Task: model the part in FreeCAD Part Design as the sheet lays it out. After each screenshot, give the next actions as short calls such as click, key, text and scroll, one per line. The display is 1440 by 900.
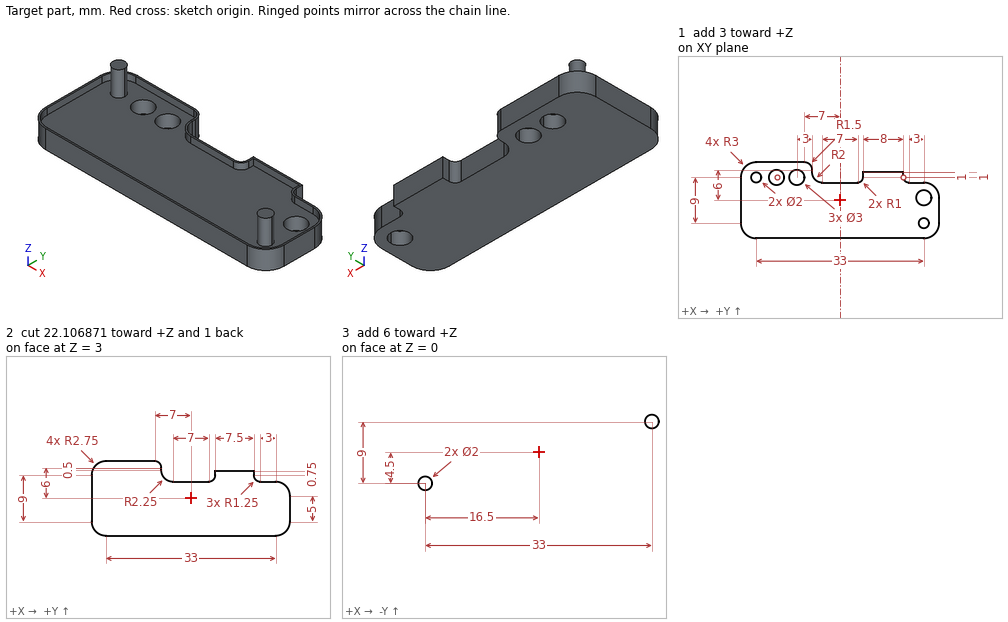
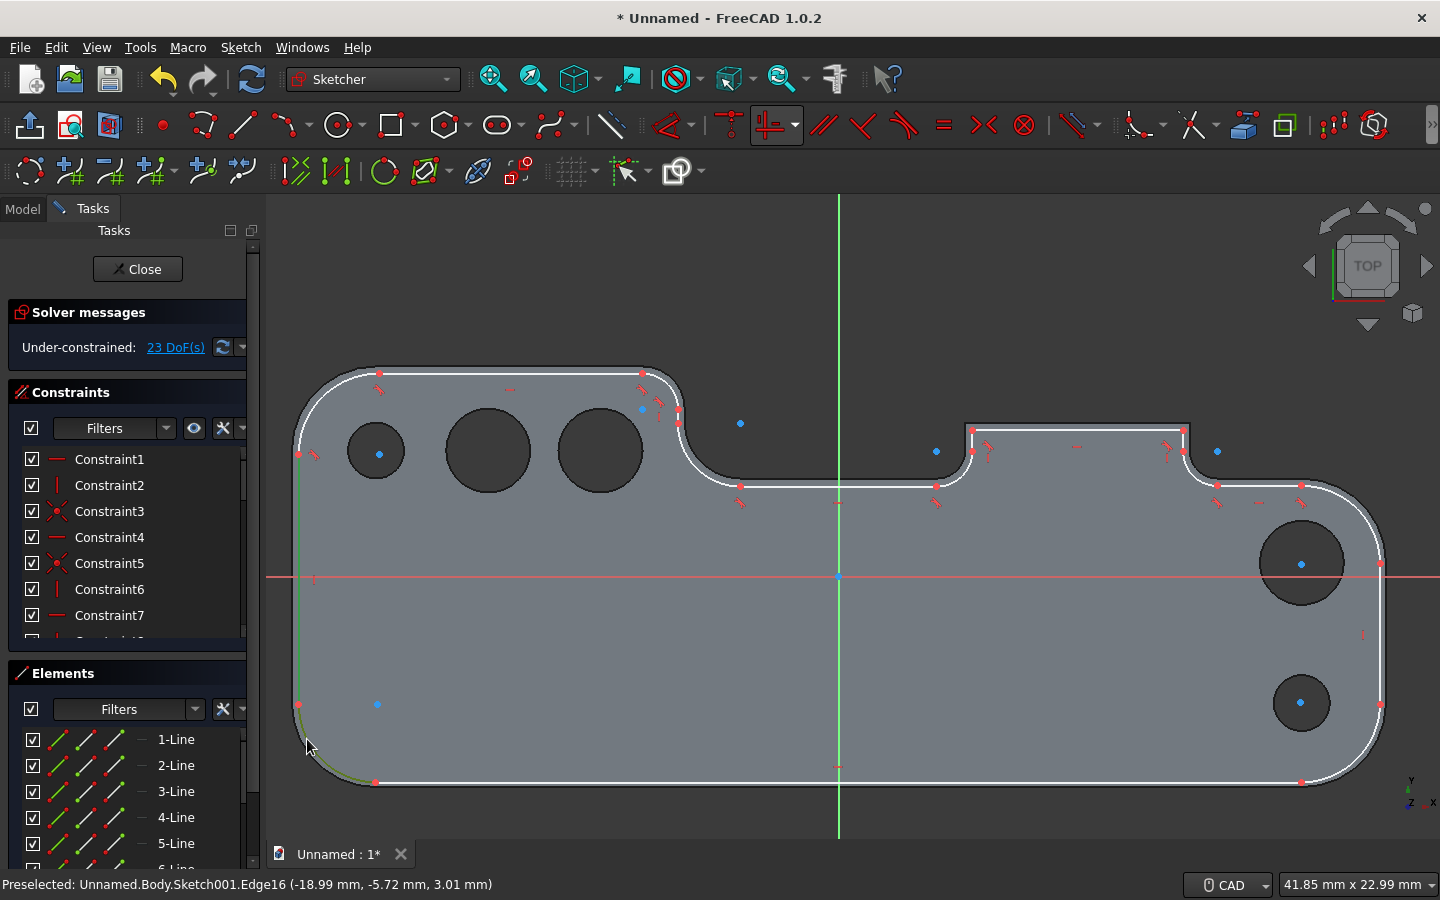
click(904, 126)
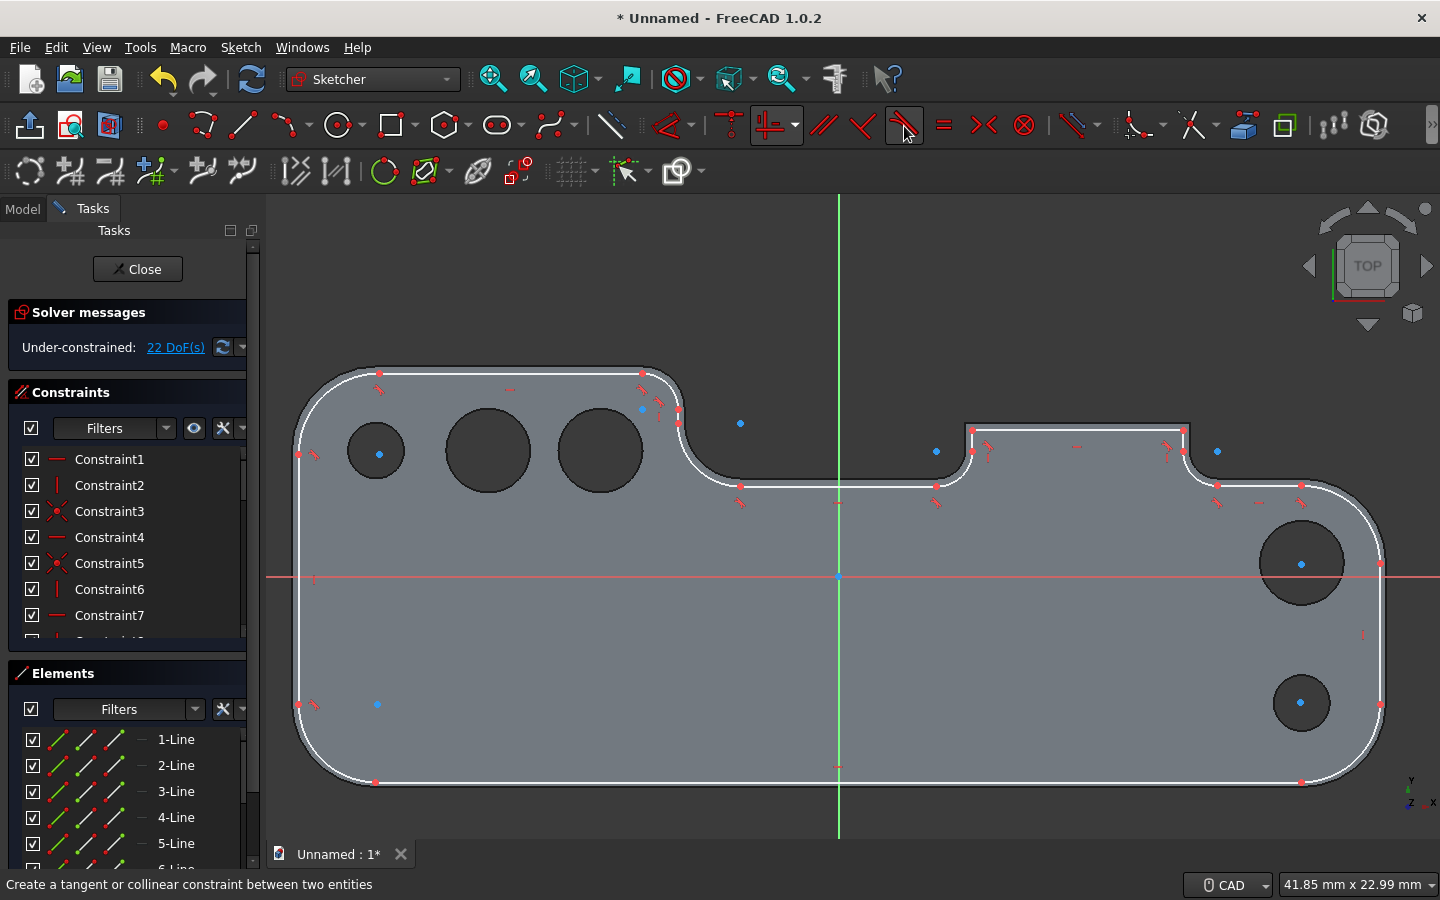
click(653, 783)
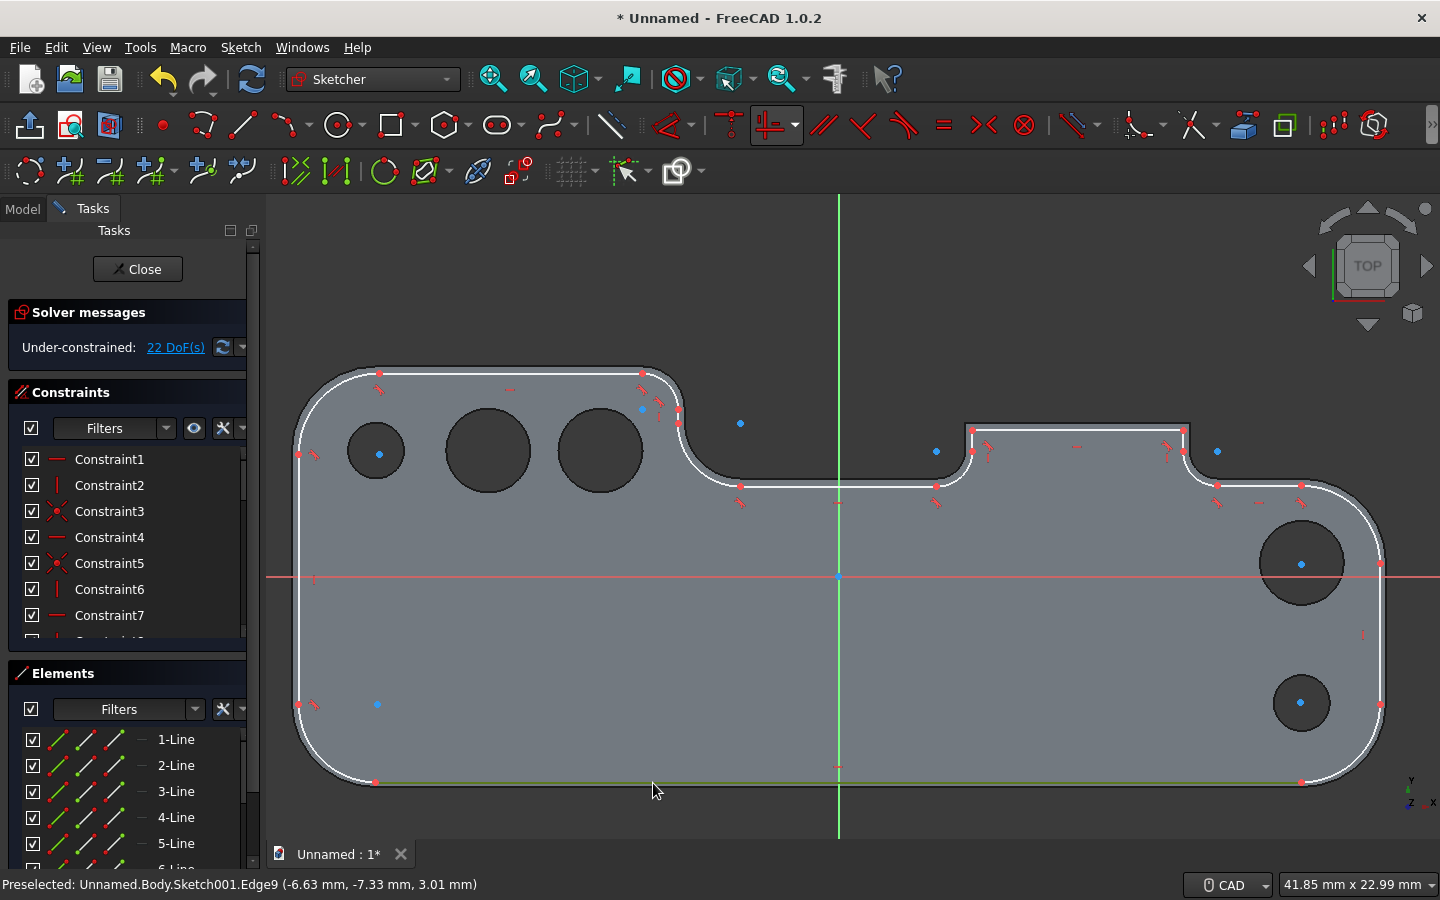
click(307, 739)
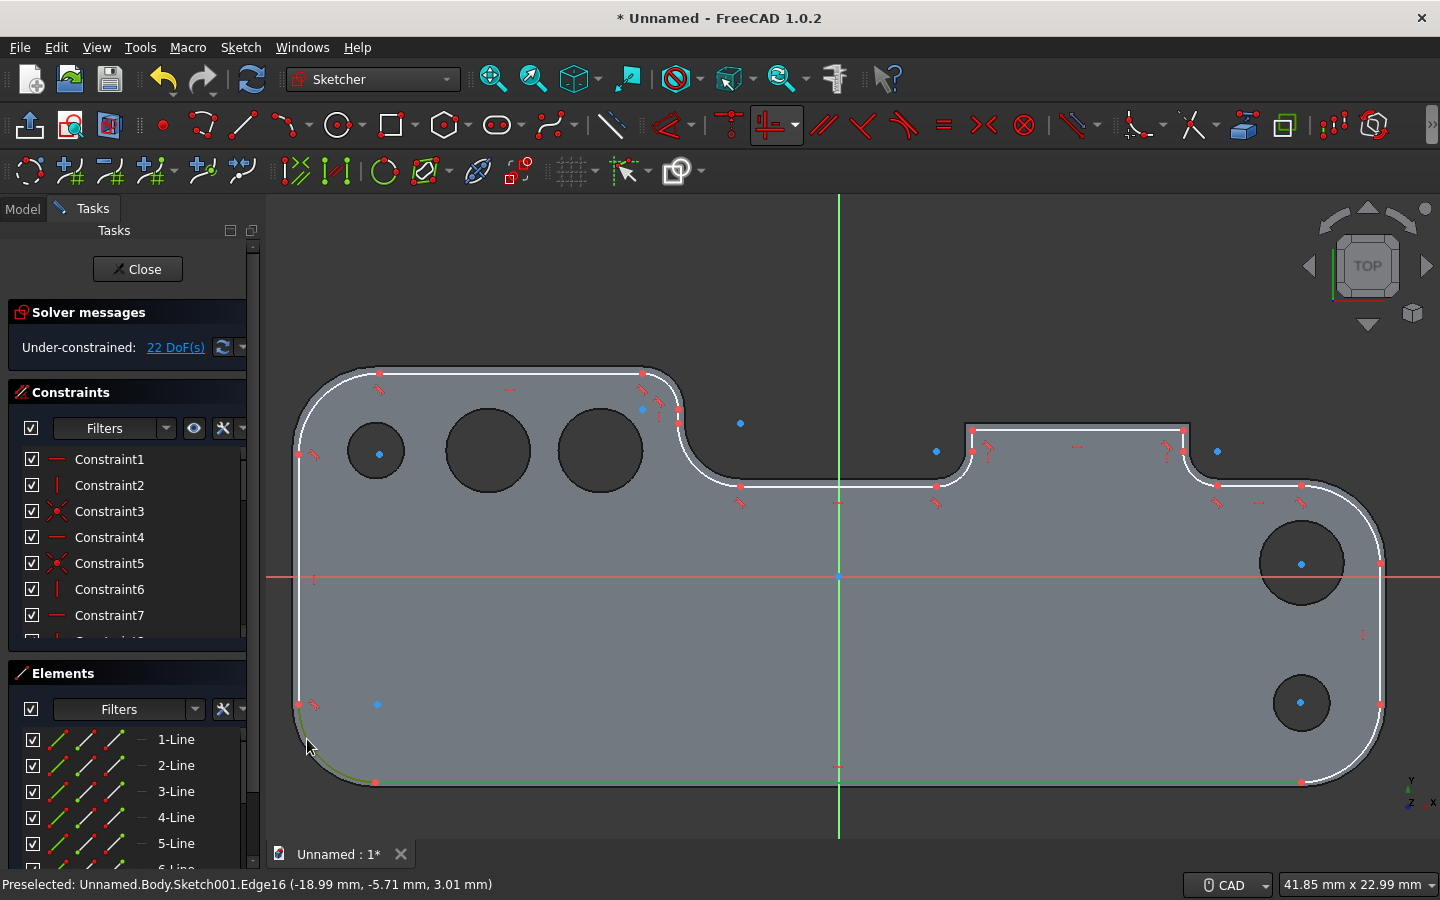
click(904, 126)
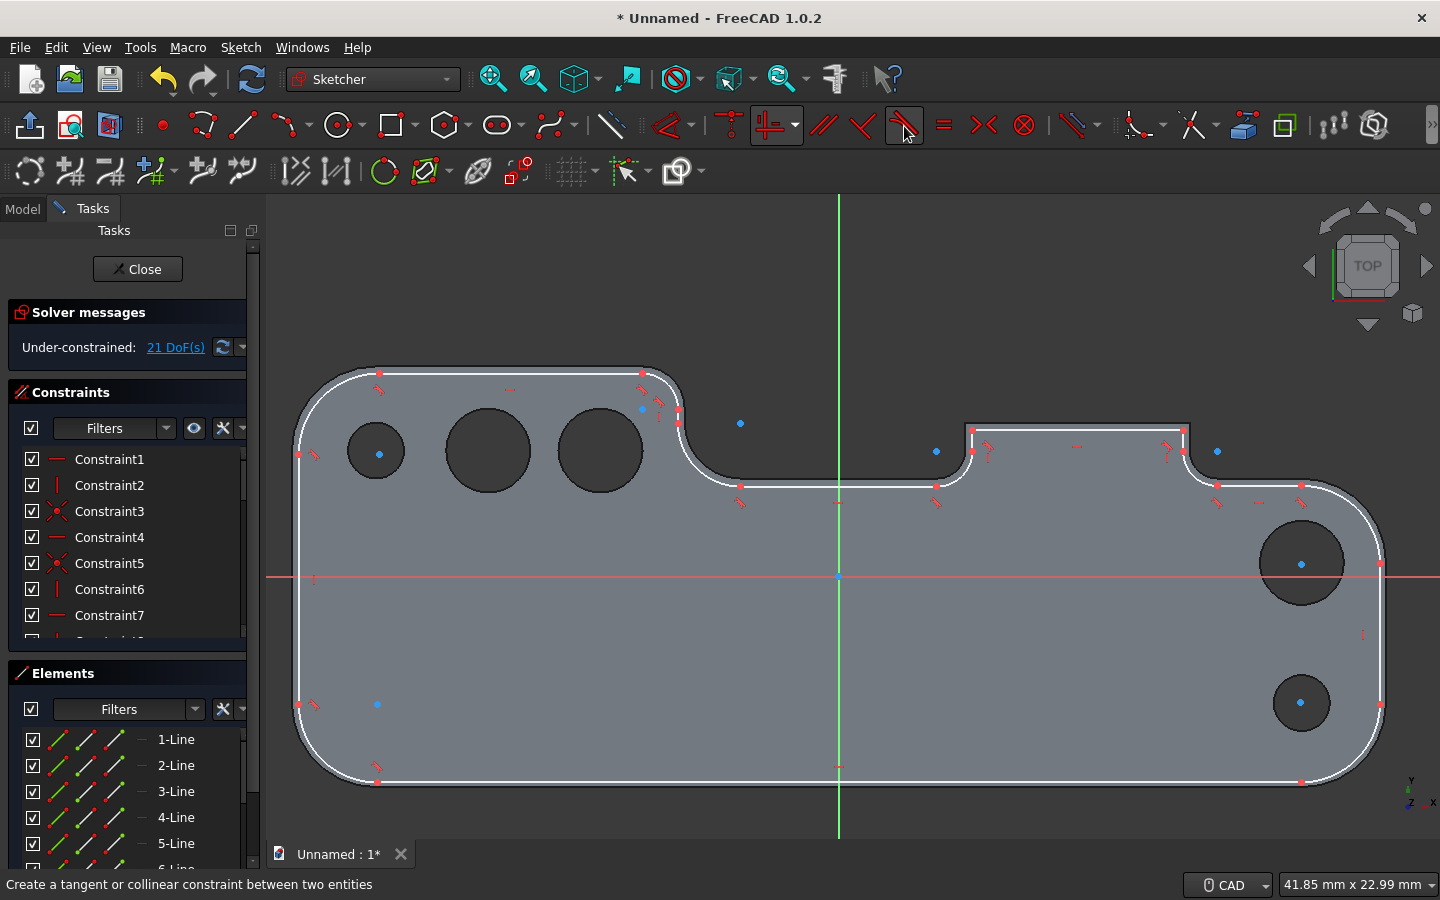
click(655, 782)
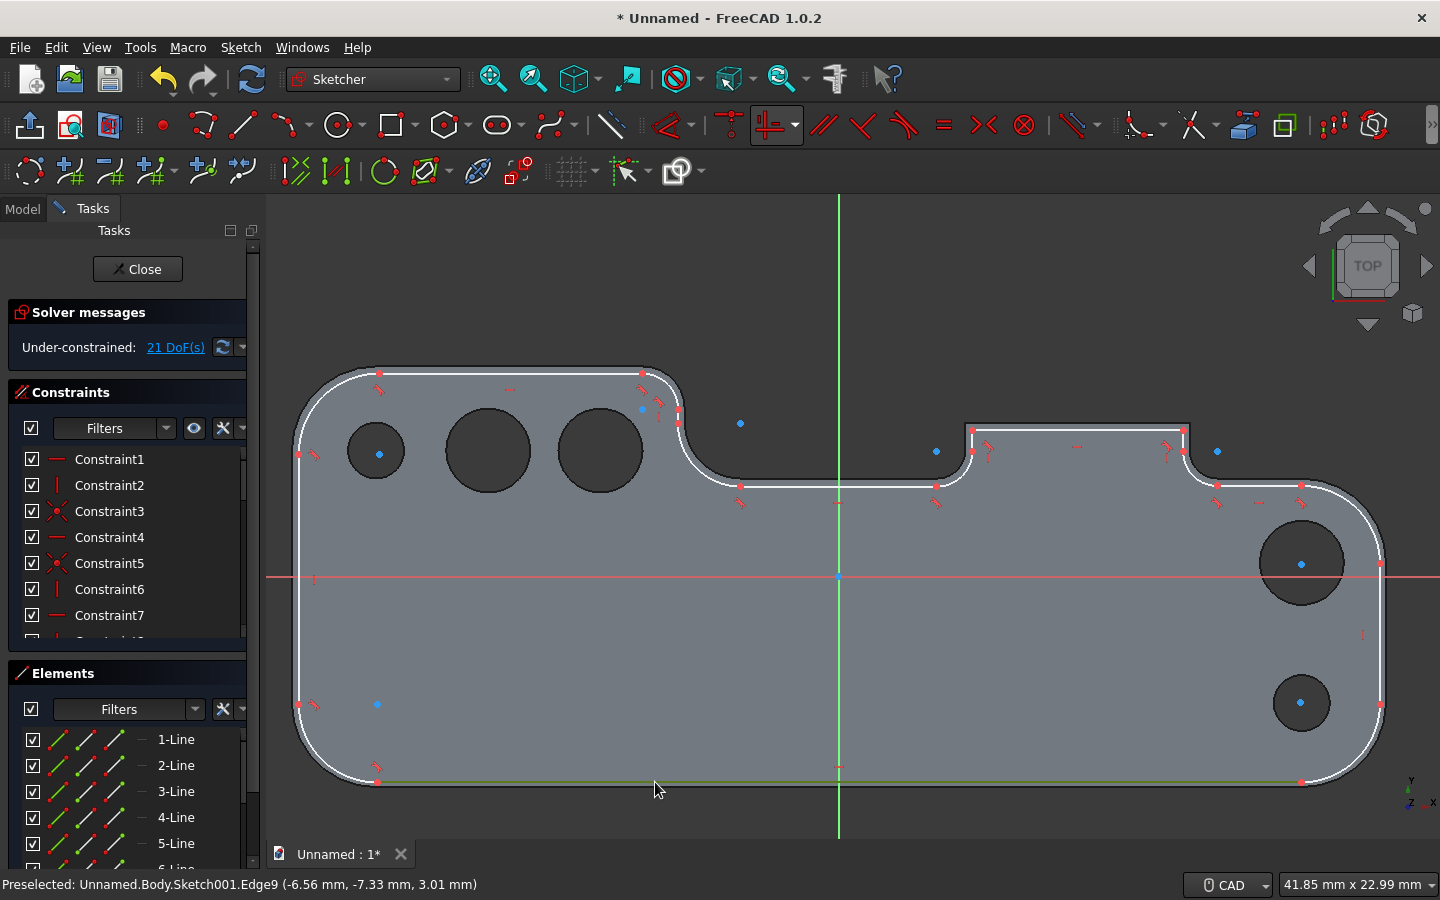
scroll(674, 394, down, 2)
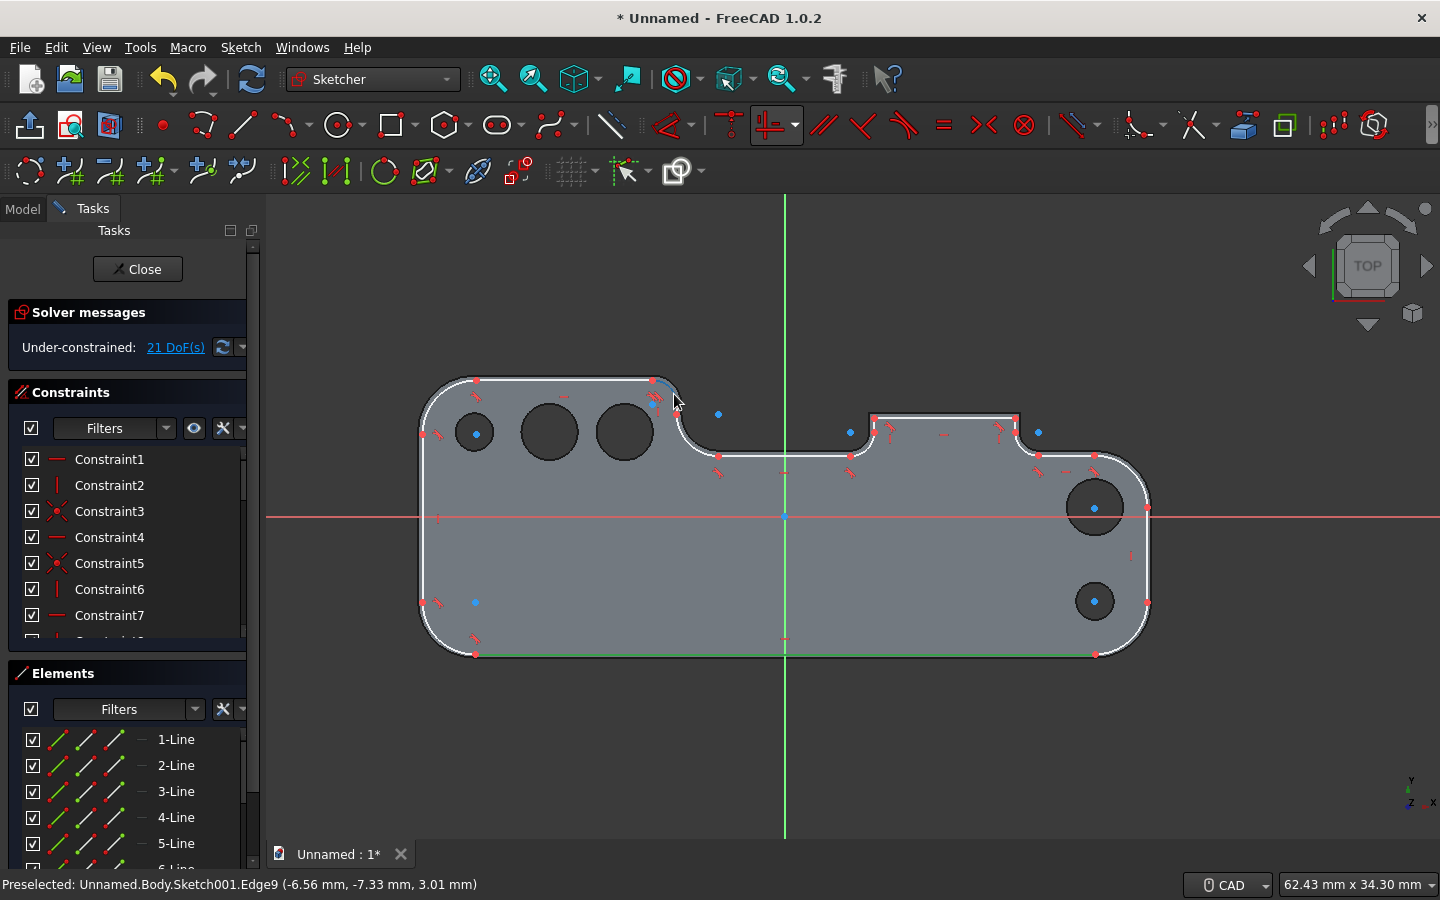
click(1119, 649)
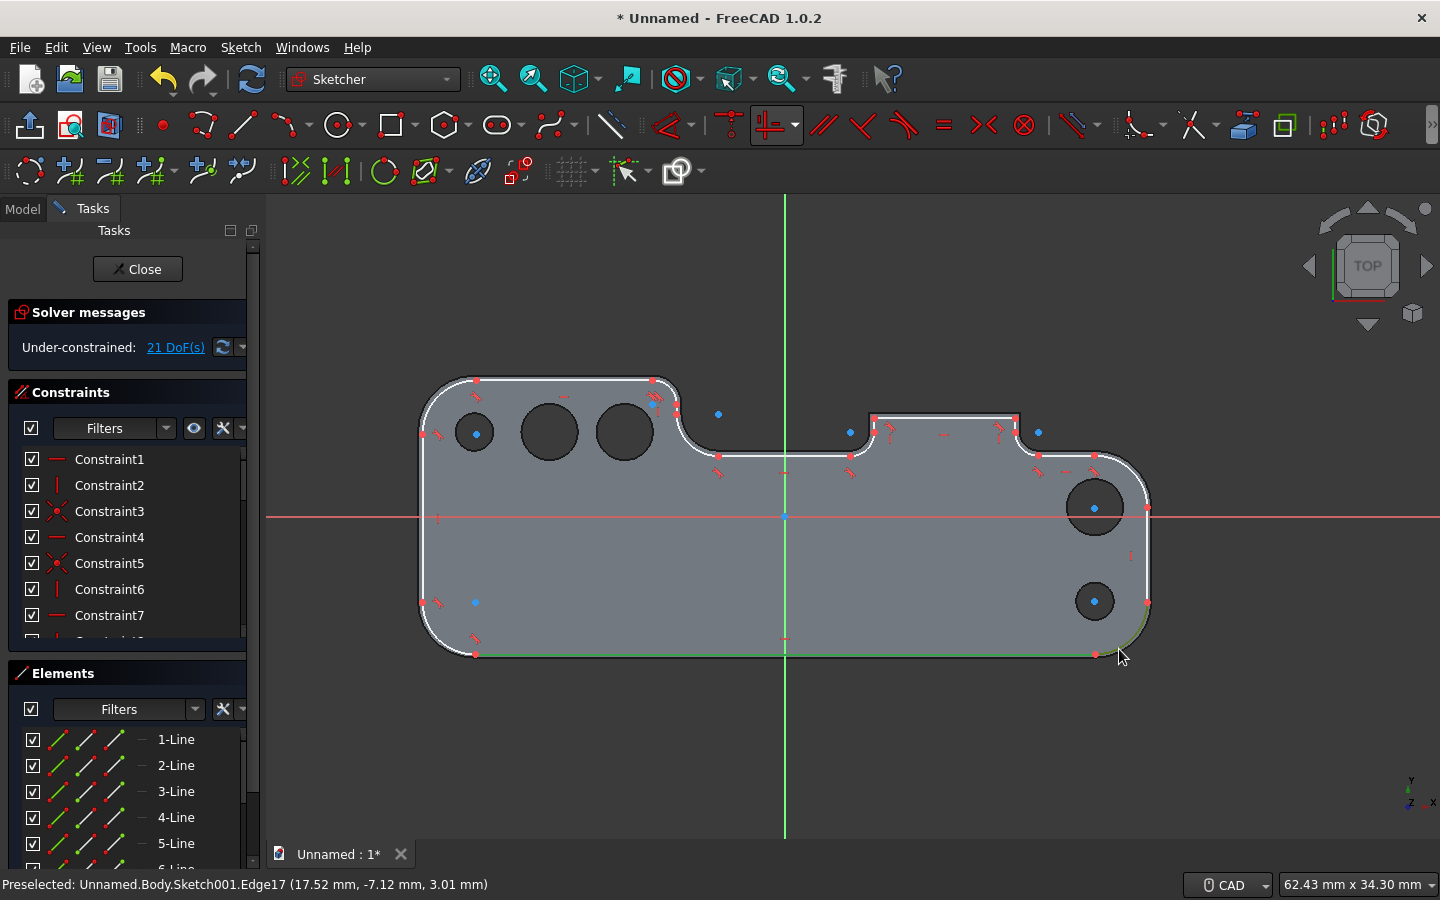
click(904, 126)